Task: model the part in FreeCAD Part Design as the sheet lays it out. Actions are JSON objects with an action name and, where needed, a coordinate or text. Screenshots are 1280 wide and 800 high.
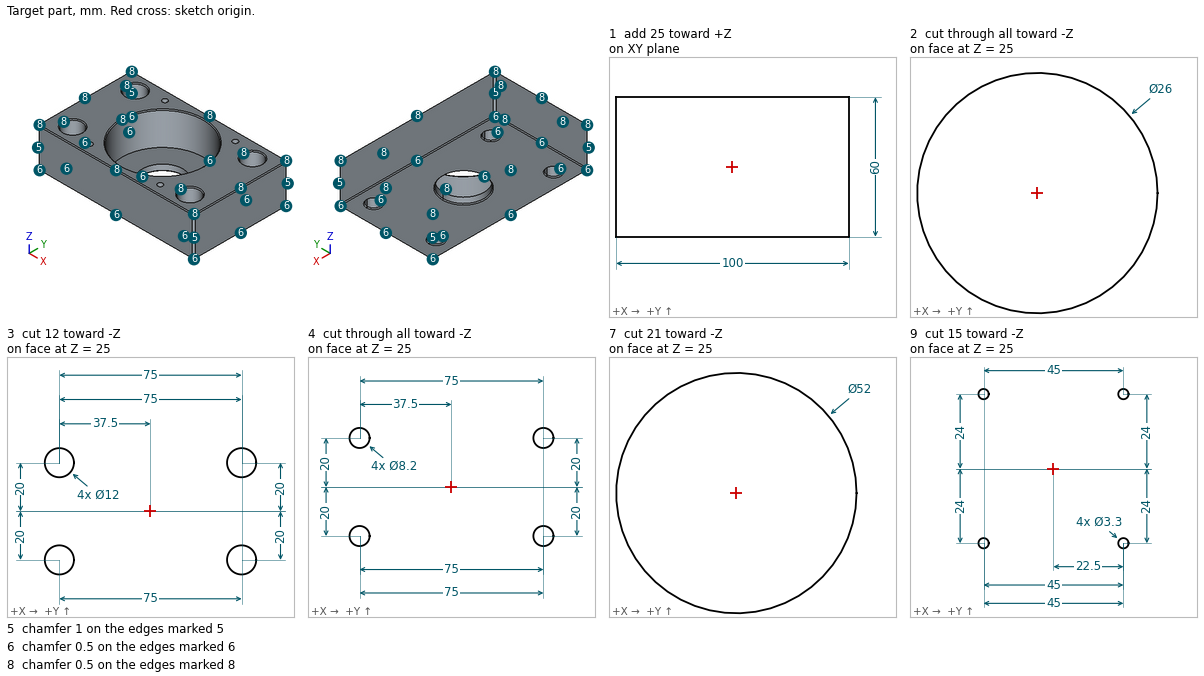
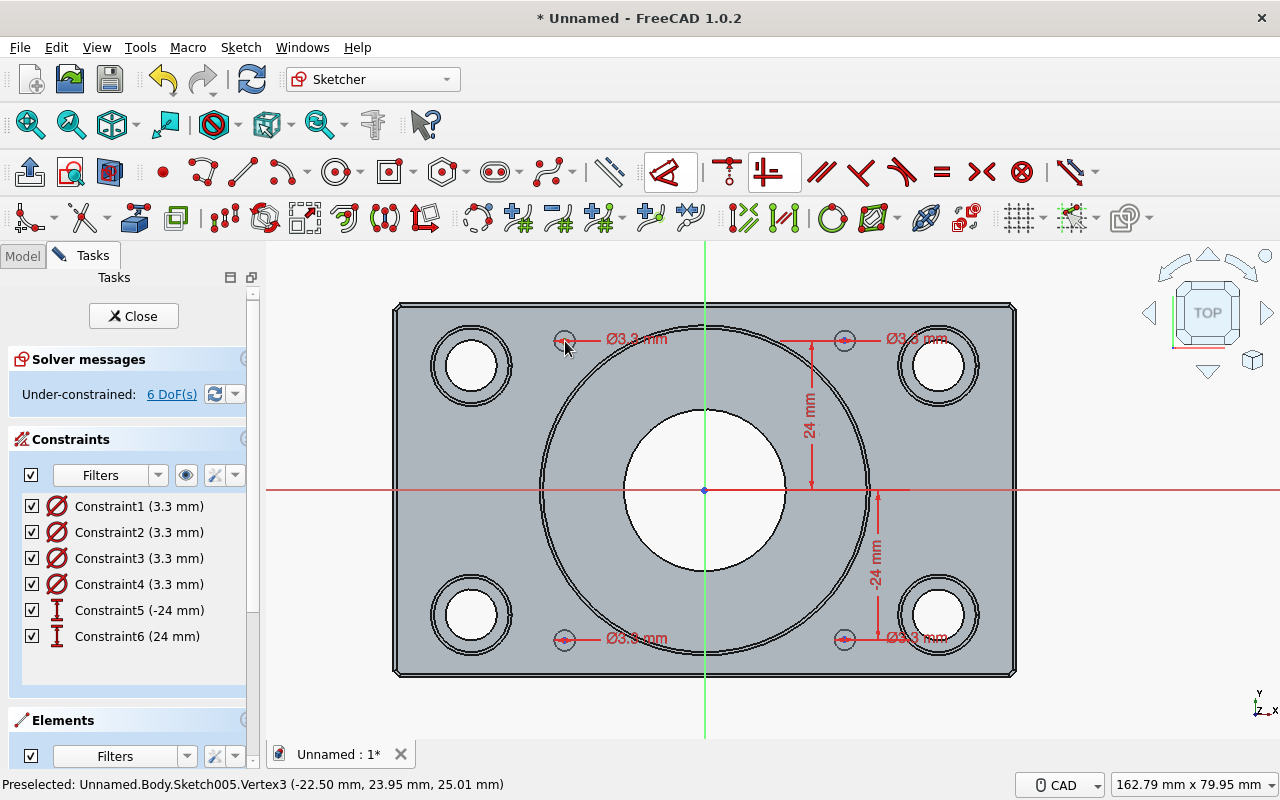
{"action": "left_click", "coordinate": [692, 172]}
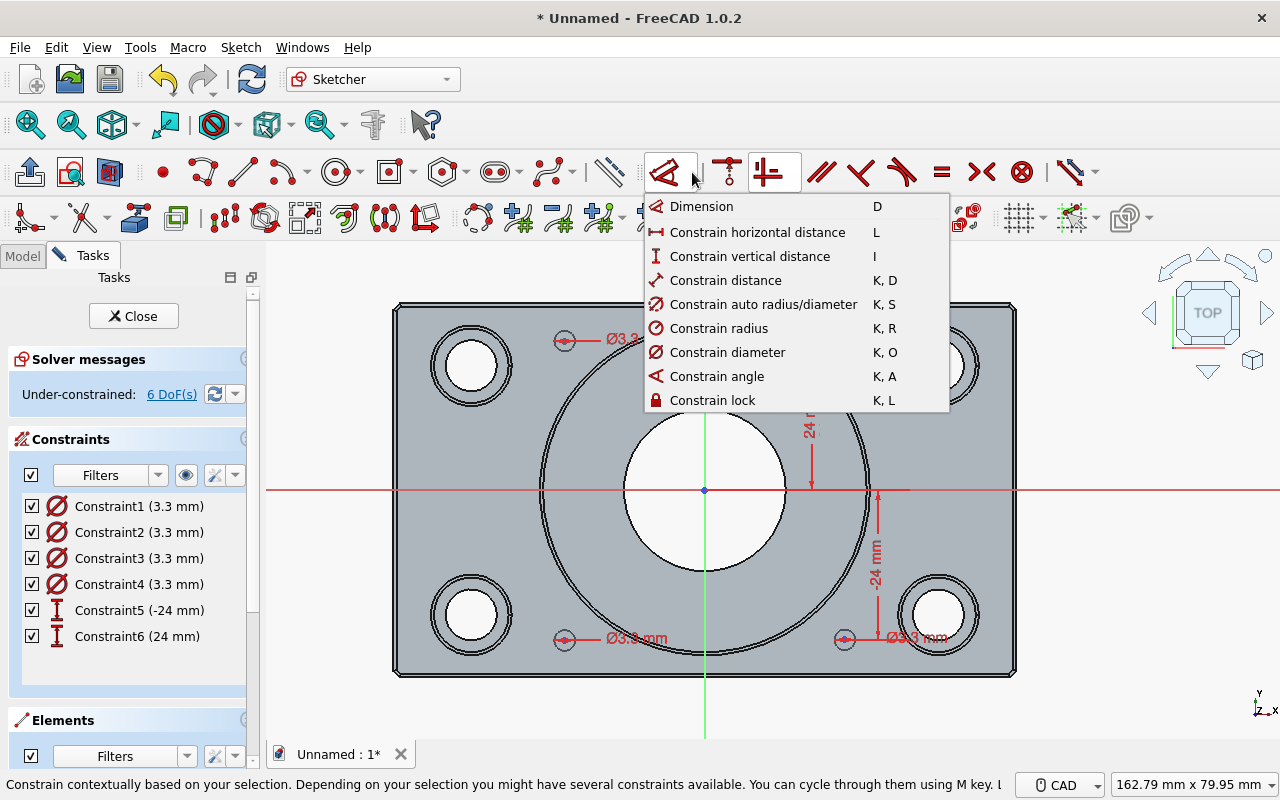
{"action": "left_click", "coordinate": [797, 256]}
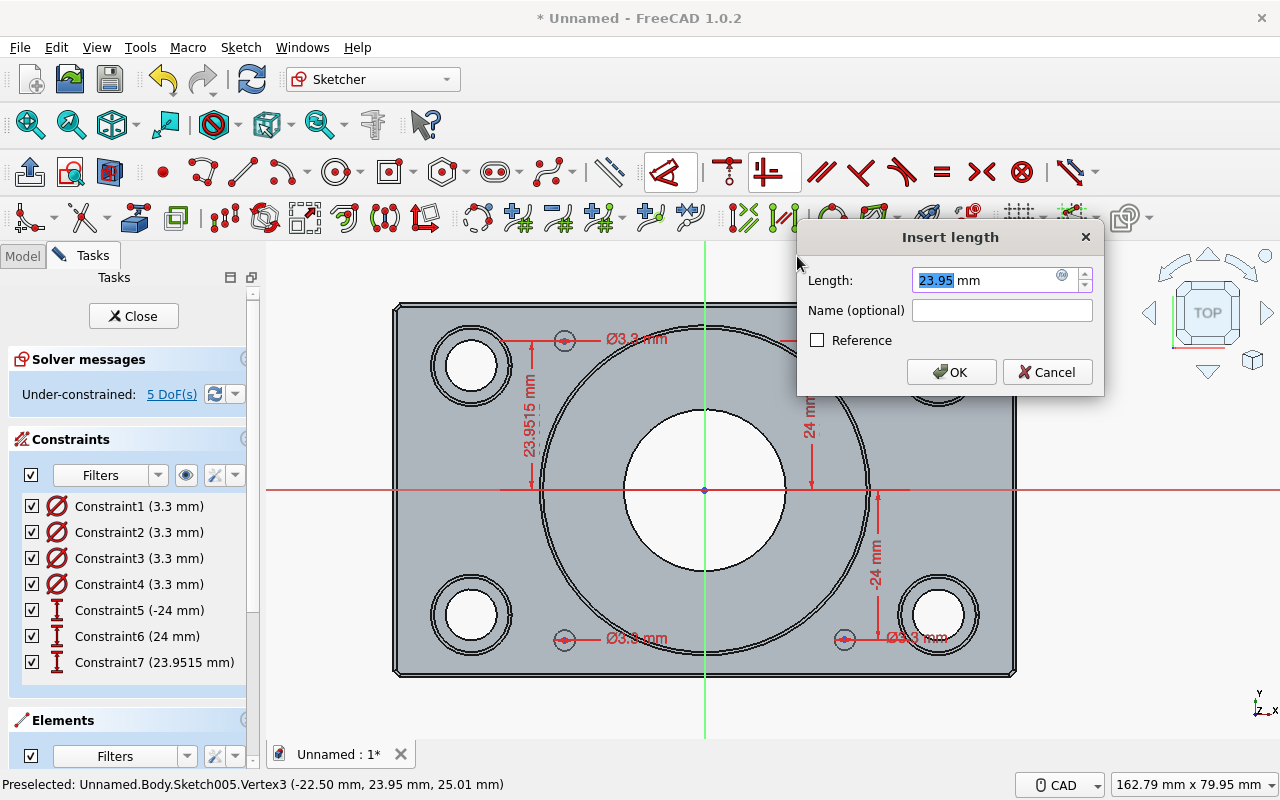
{"action": "type", "text": "24"}
{"action": "key", "text": "Return"}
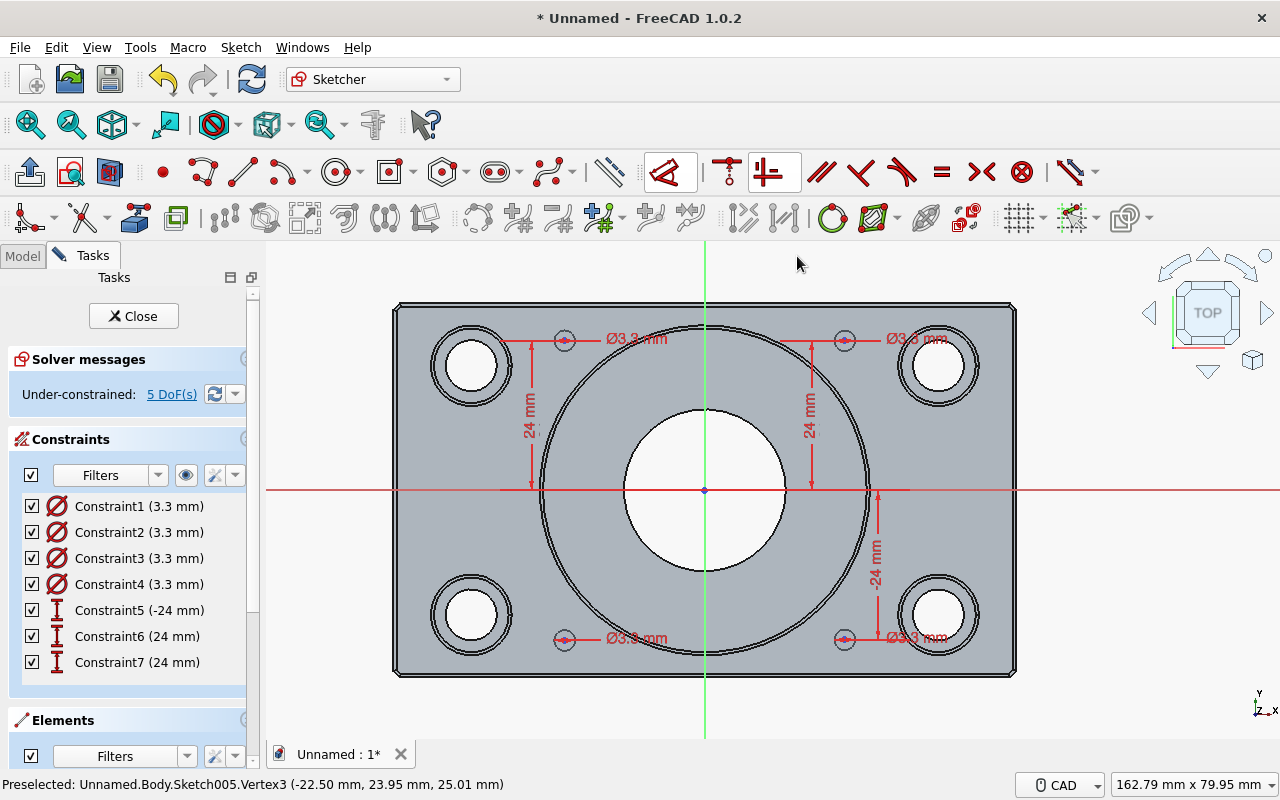
{"action": "left_click", "coordinate": [565, 640]}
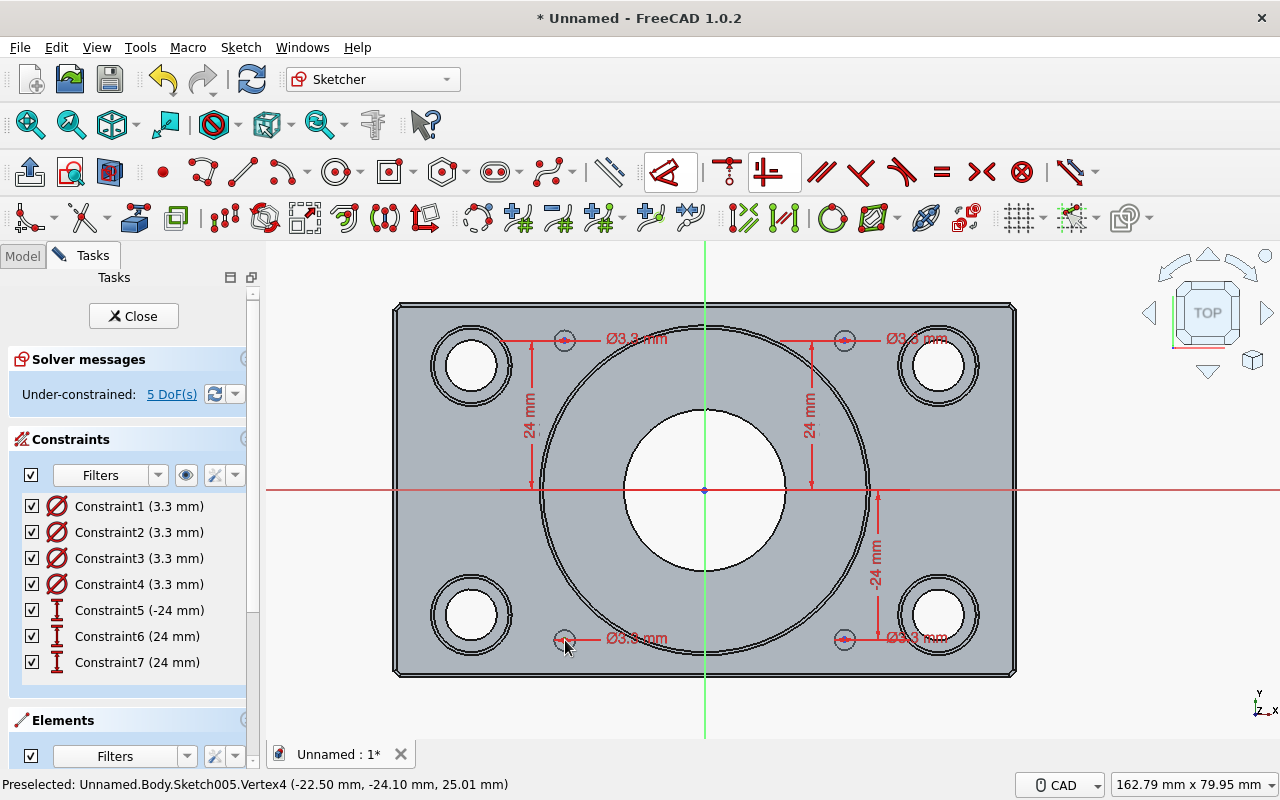
{"action": "key", "text": "i"}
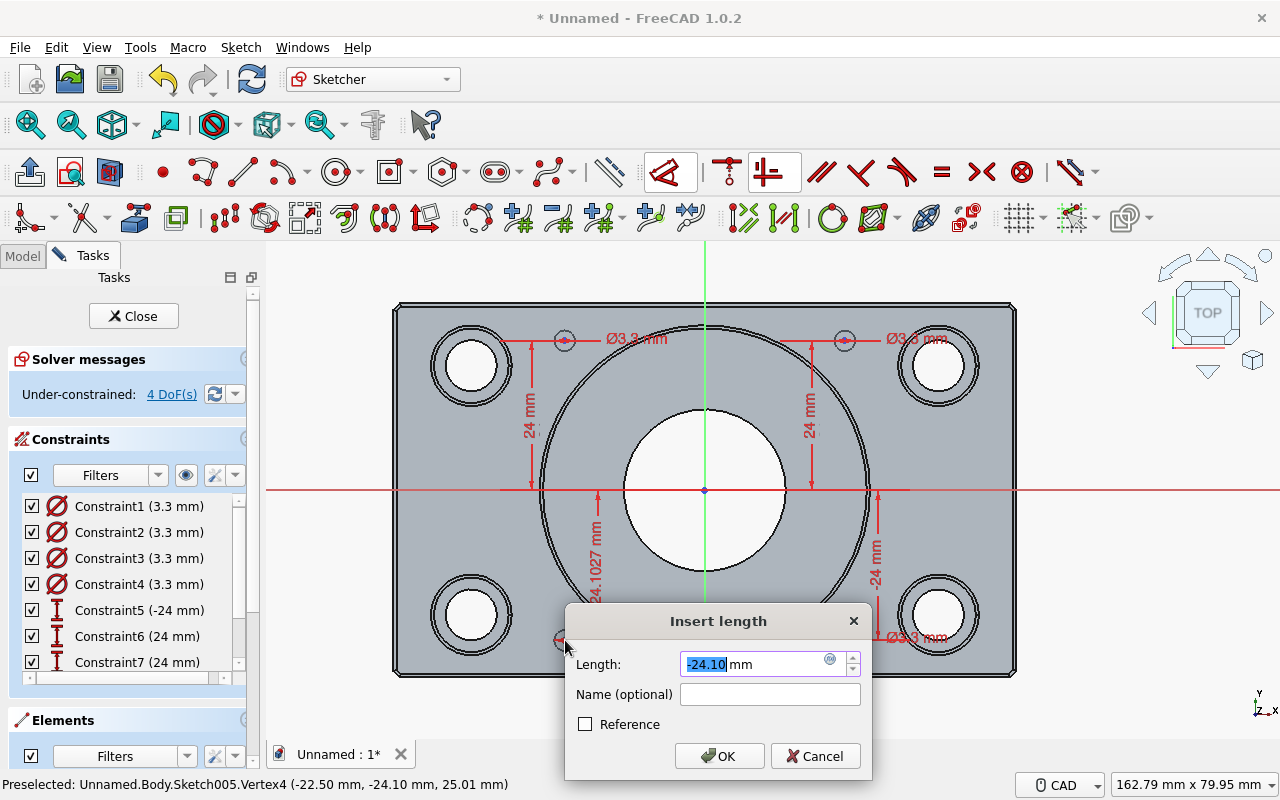
{"action": "type", "text": "-24"}
{"action": "key", "text": "Return"}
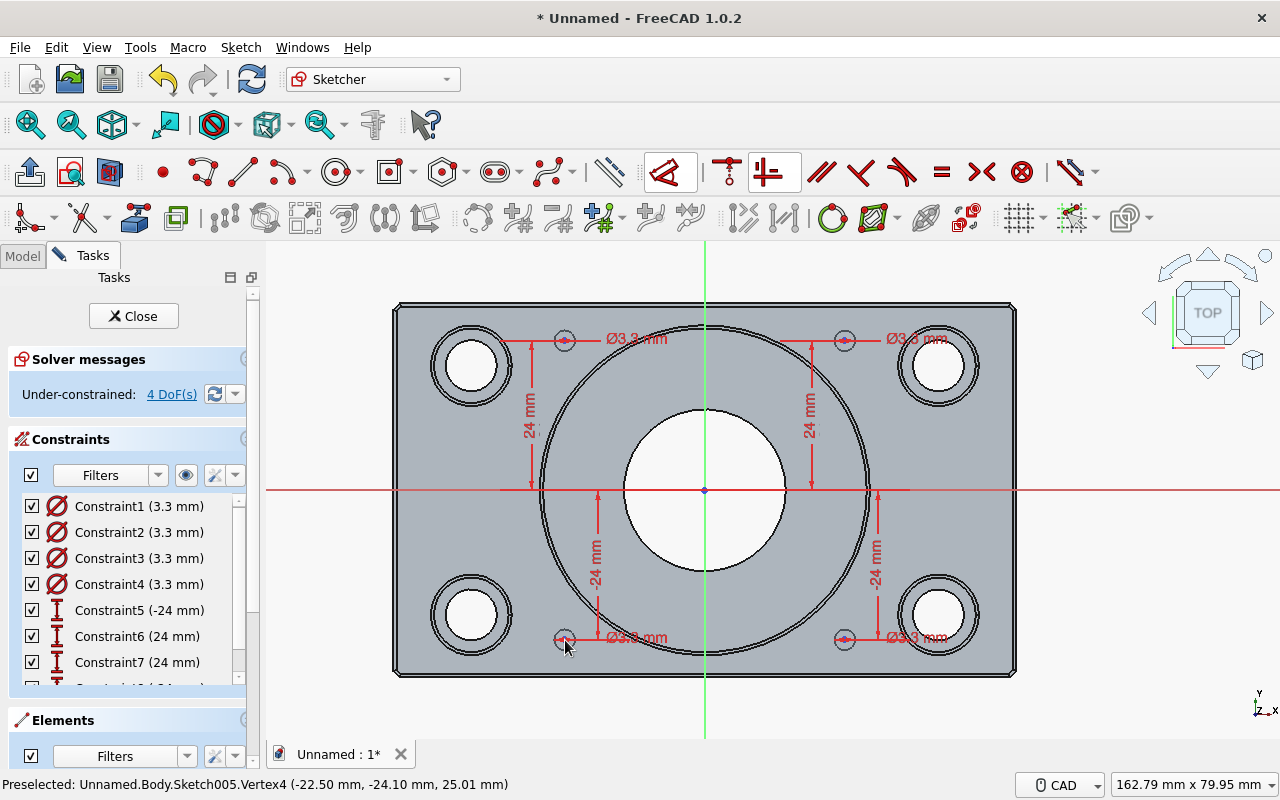
{"action": "left_click", "coordinate": [845, 341]}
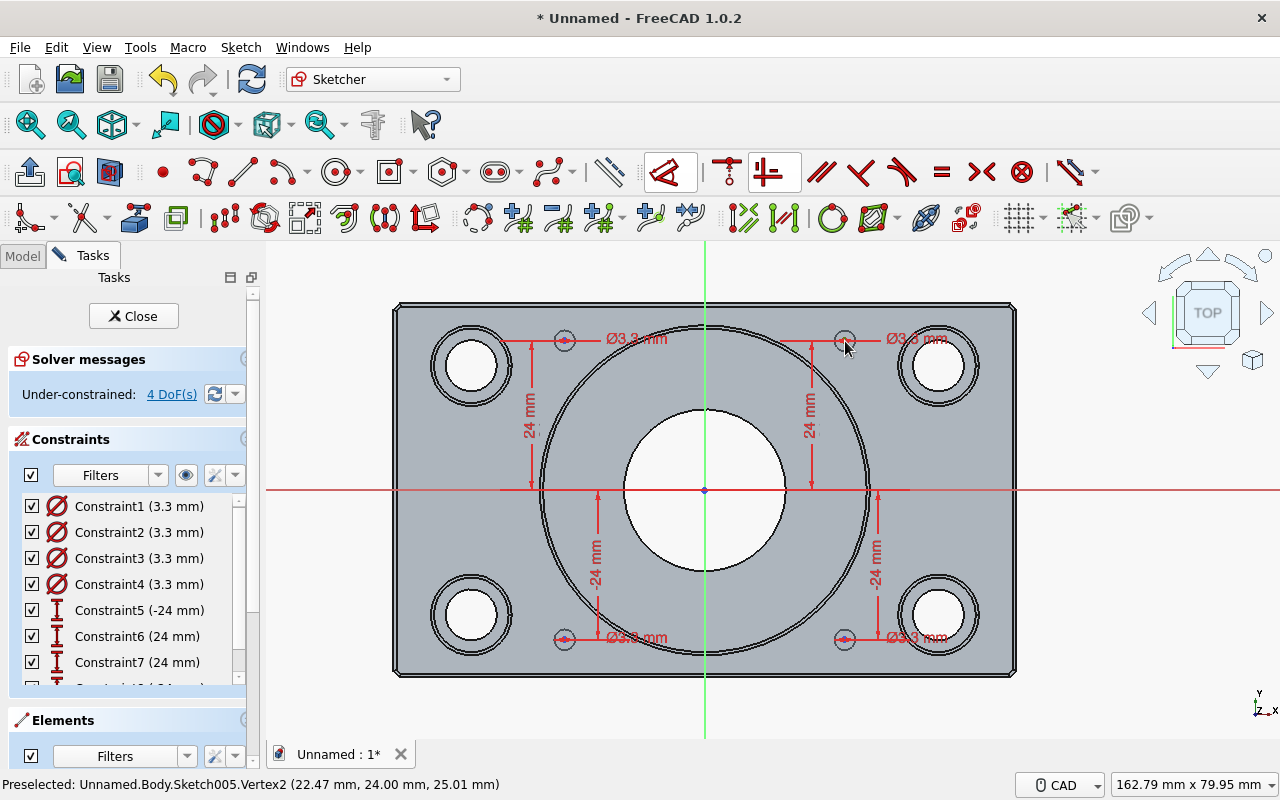
{"action": "left_click", "coordinate": [565, 341]}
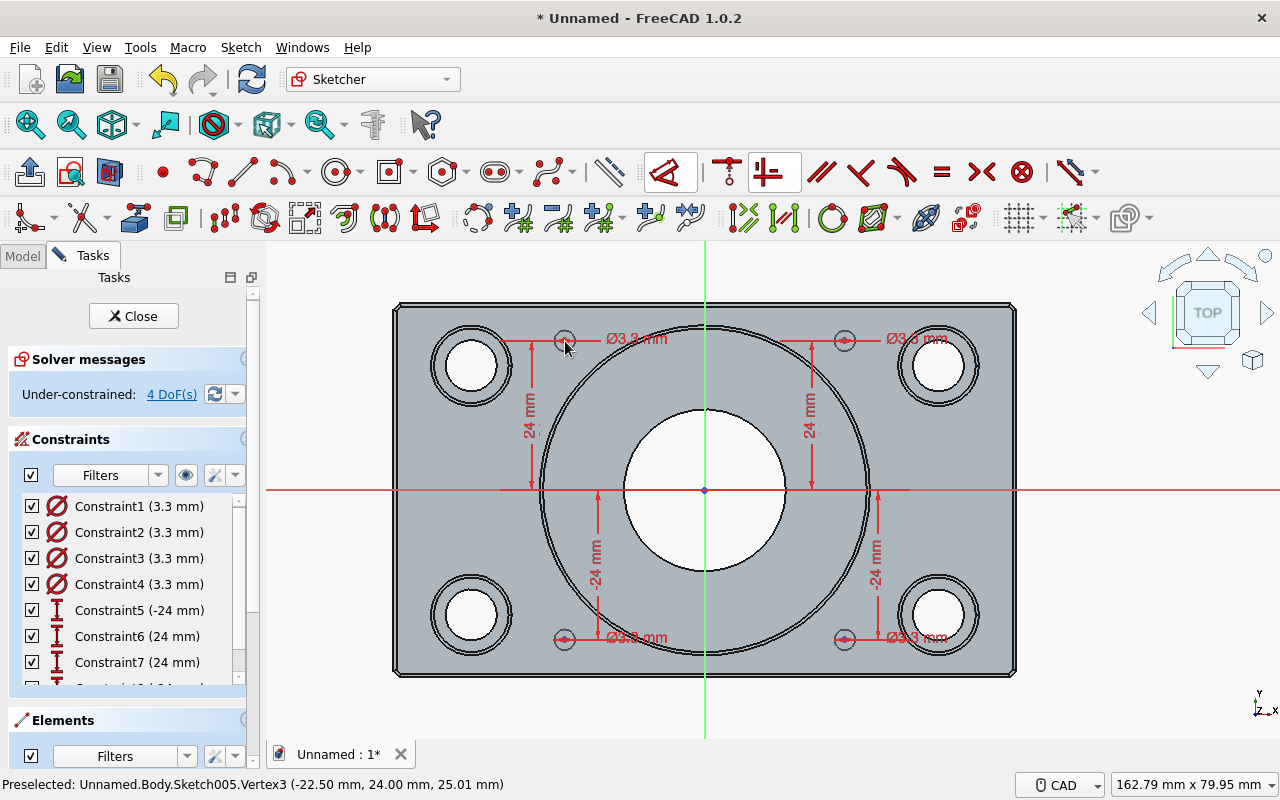
{"action": "left_click", "coordinate": [692, 172]}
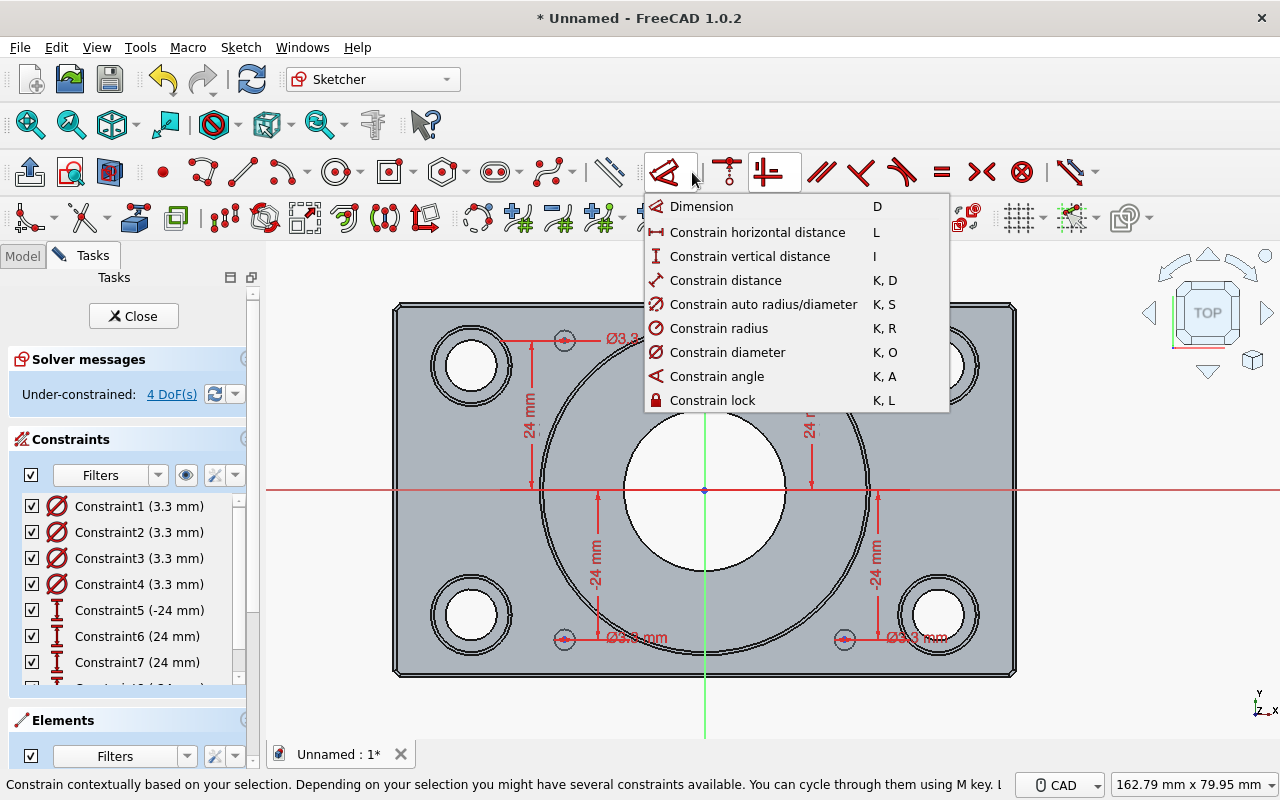
{"action": "left_click", "coordinate": [797, 232]}